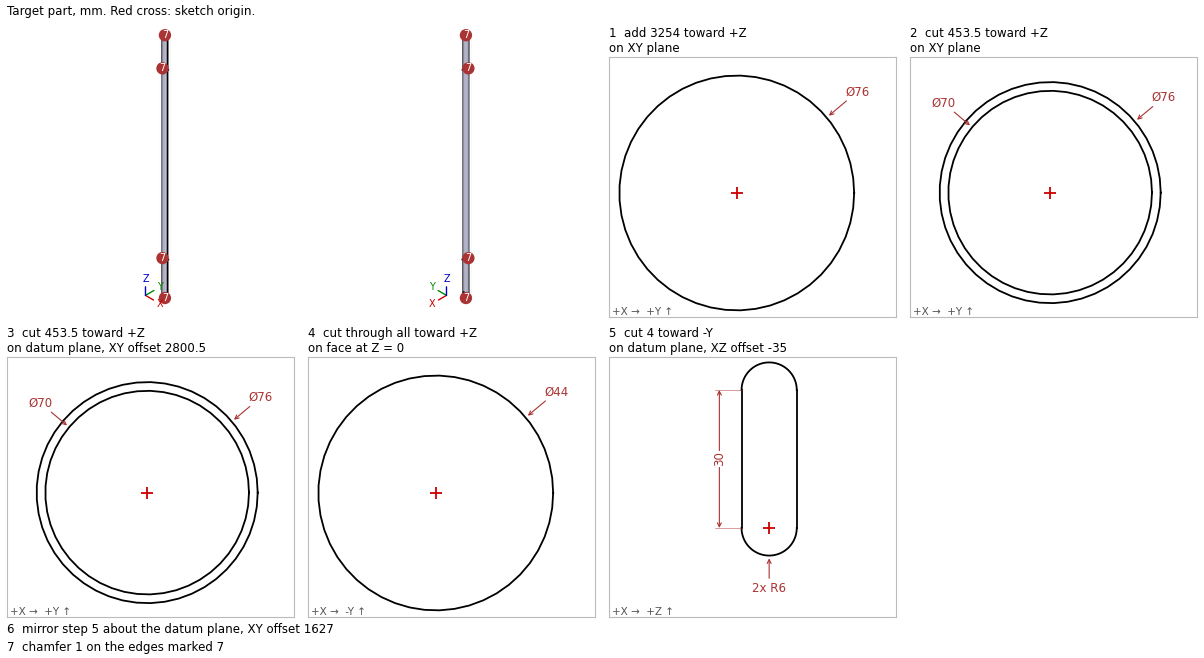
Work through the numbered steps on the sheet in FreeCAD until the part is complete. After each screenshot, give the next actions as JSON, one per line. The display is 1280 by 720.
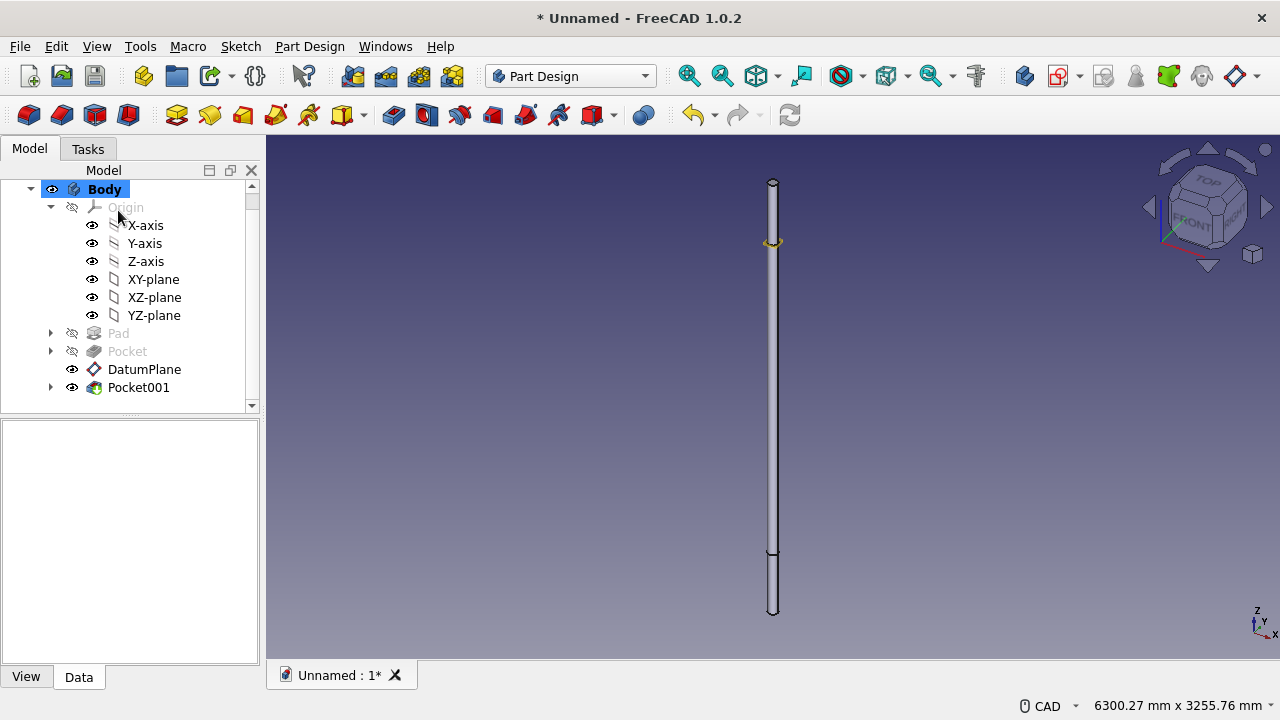
{"action": "left_click", "coordinate": [117, 369]}
{"action": "key", "text": "space"}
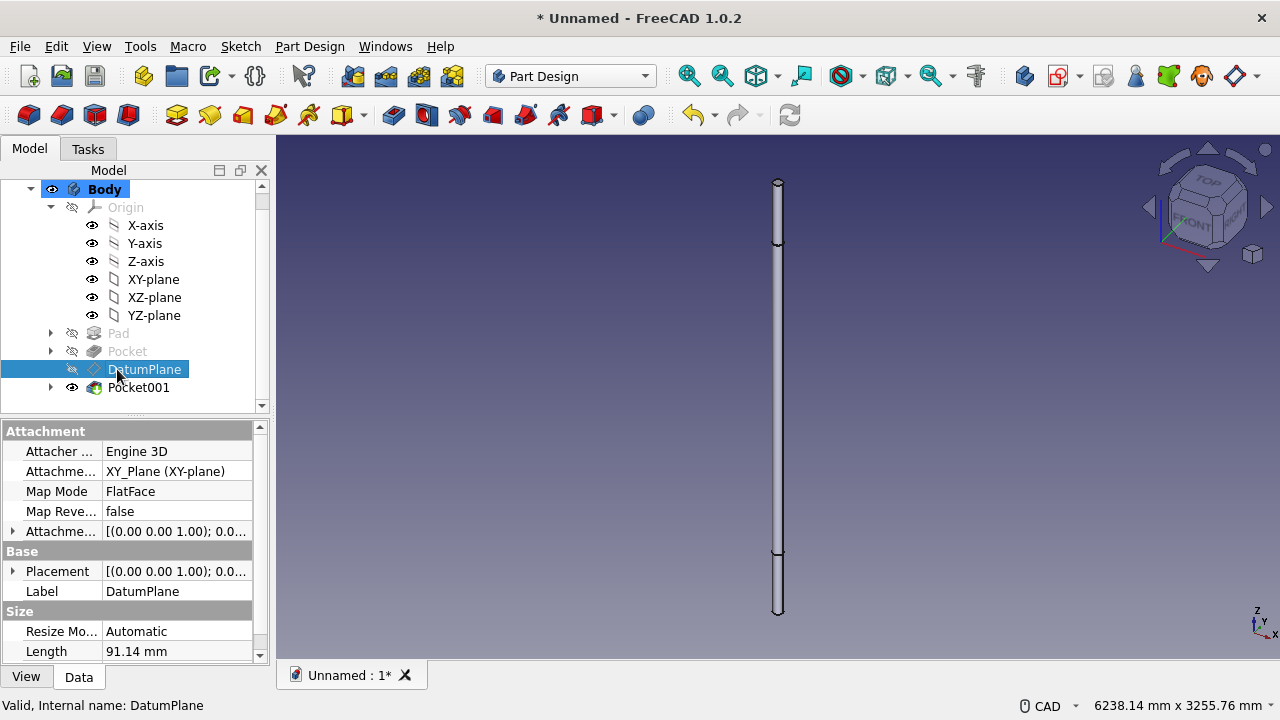
{"action": "key", "text": "5"}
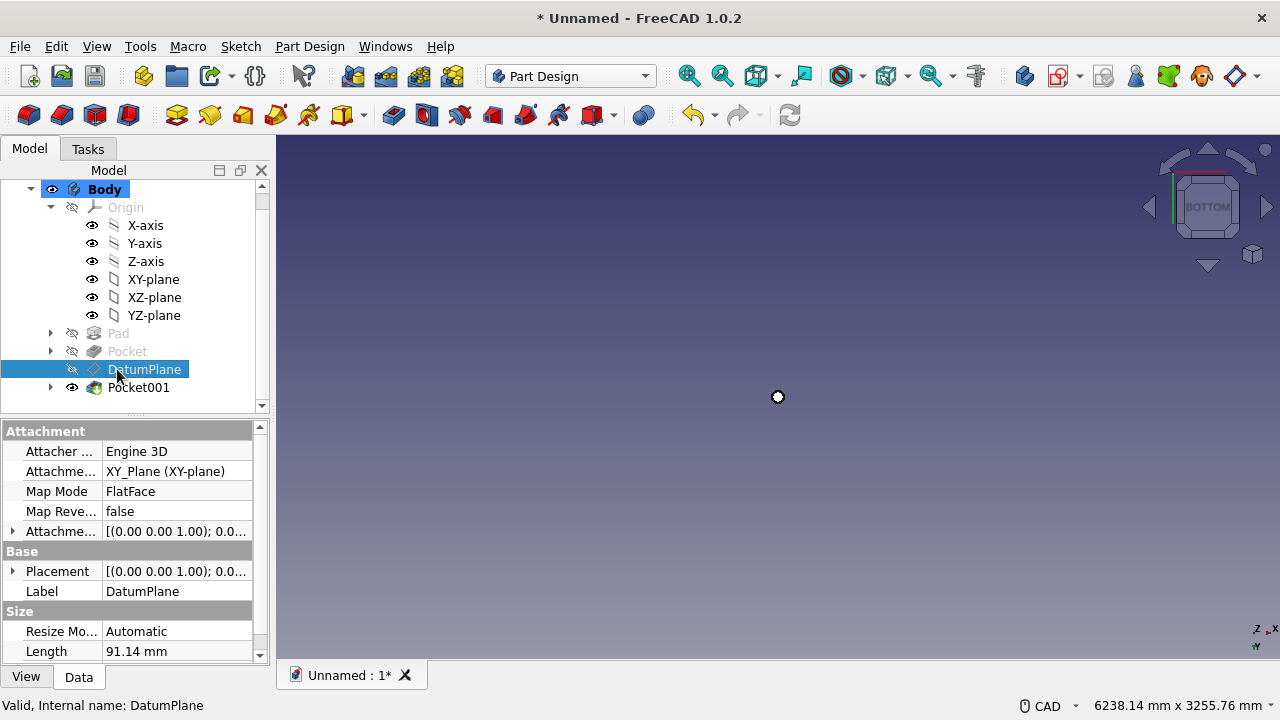
{"action": "left_click", "coordinate": [690, 76]}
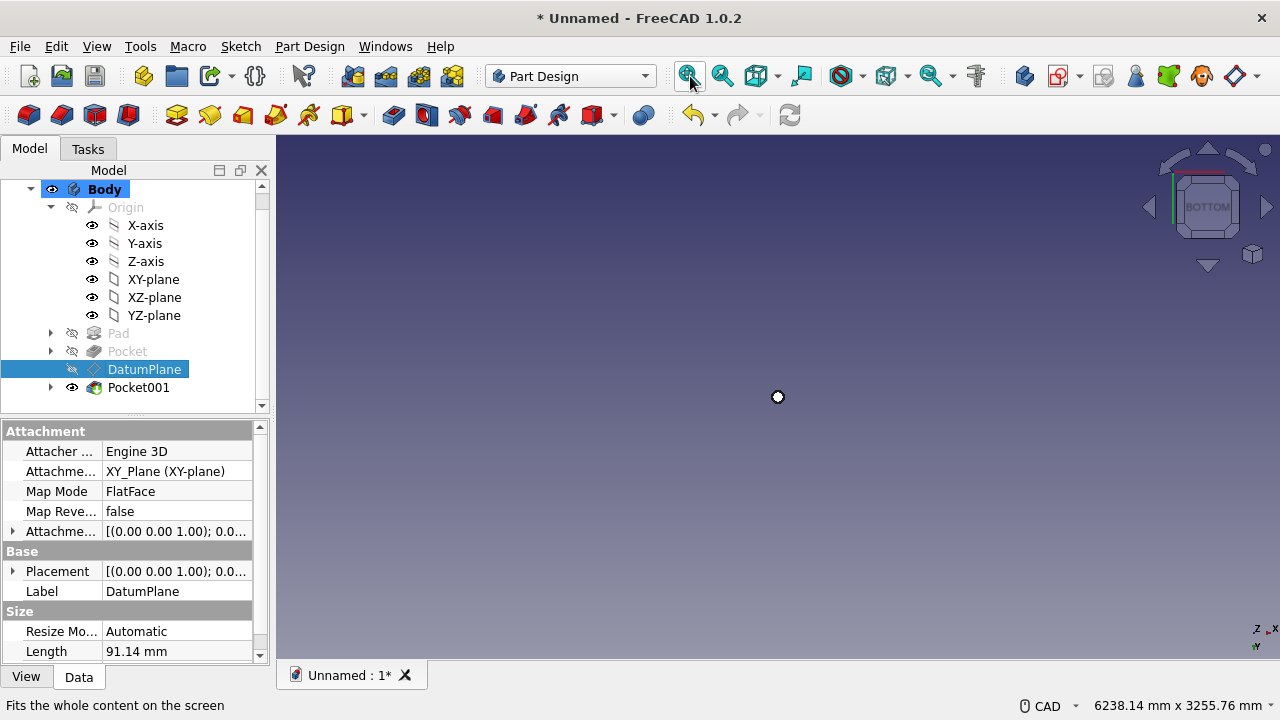
{"action": "scroll", "coordinate": [778, 396], "scroll_direction": "up", "scroll_amount": 4}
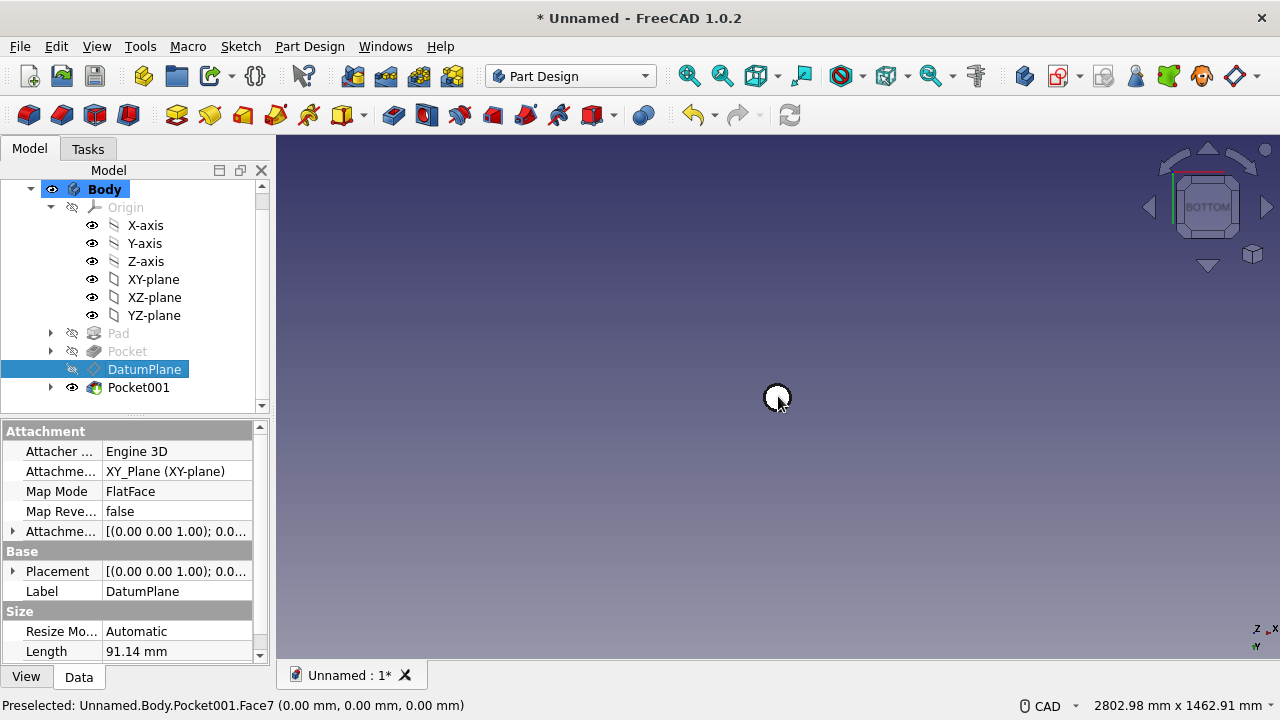
{"action": "left_click", "coordinate": [777, 397]}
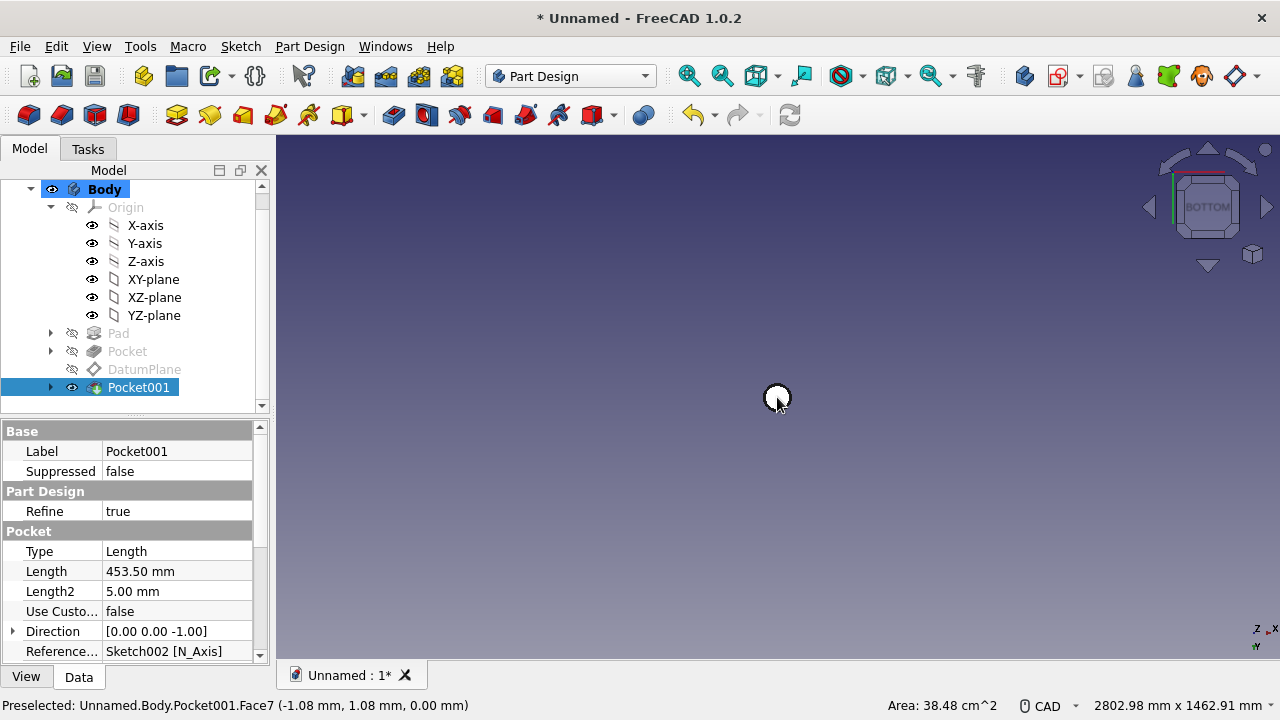
{"action": "left_click", "coordinate": [1058, 76]}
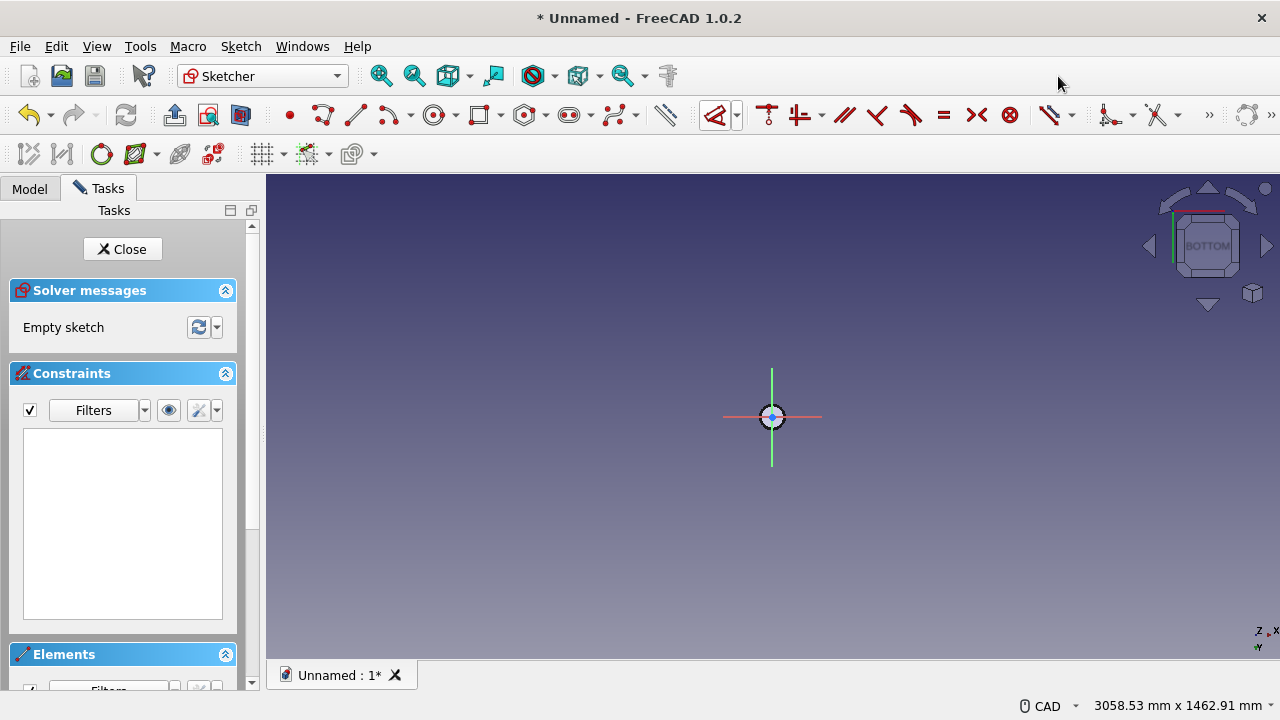
{"action": "scroll", "coordinate": [776, 417], "scroll_direction": "up", "scroll_amount": 15}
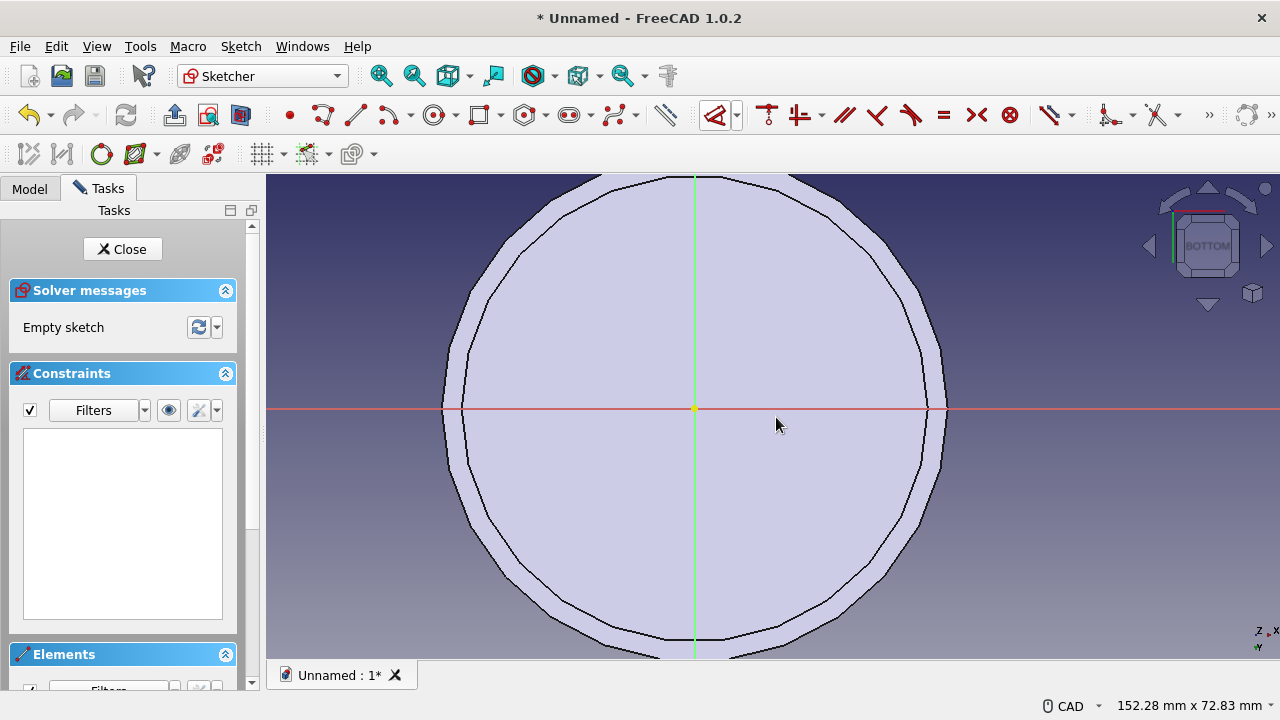
{"action": "left_click", "coordinate": [434, 116]}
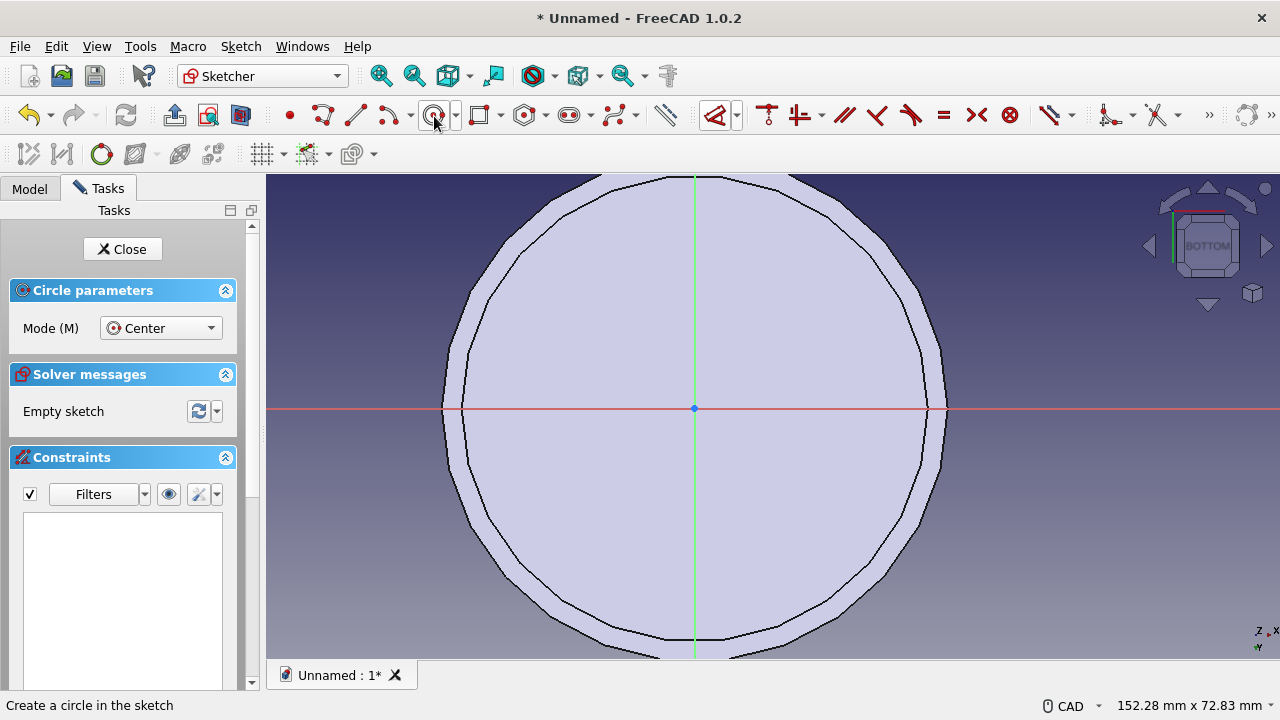
{"action": "left_click", "coordinate": [695, 409]}
{"action": "left_click", "coordinate": [798, 305]}
{"action": "key", "text": "Escape"}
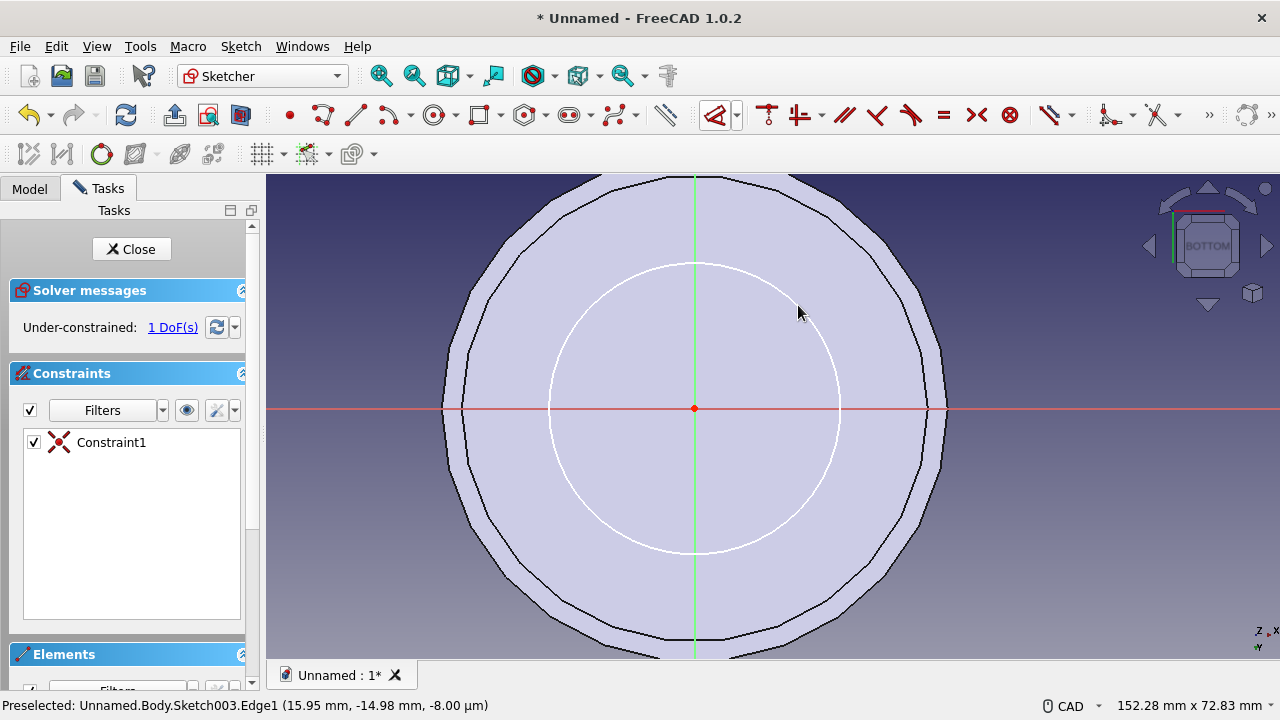
{"action": "left_click", "coordinate": [797, 305]}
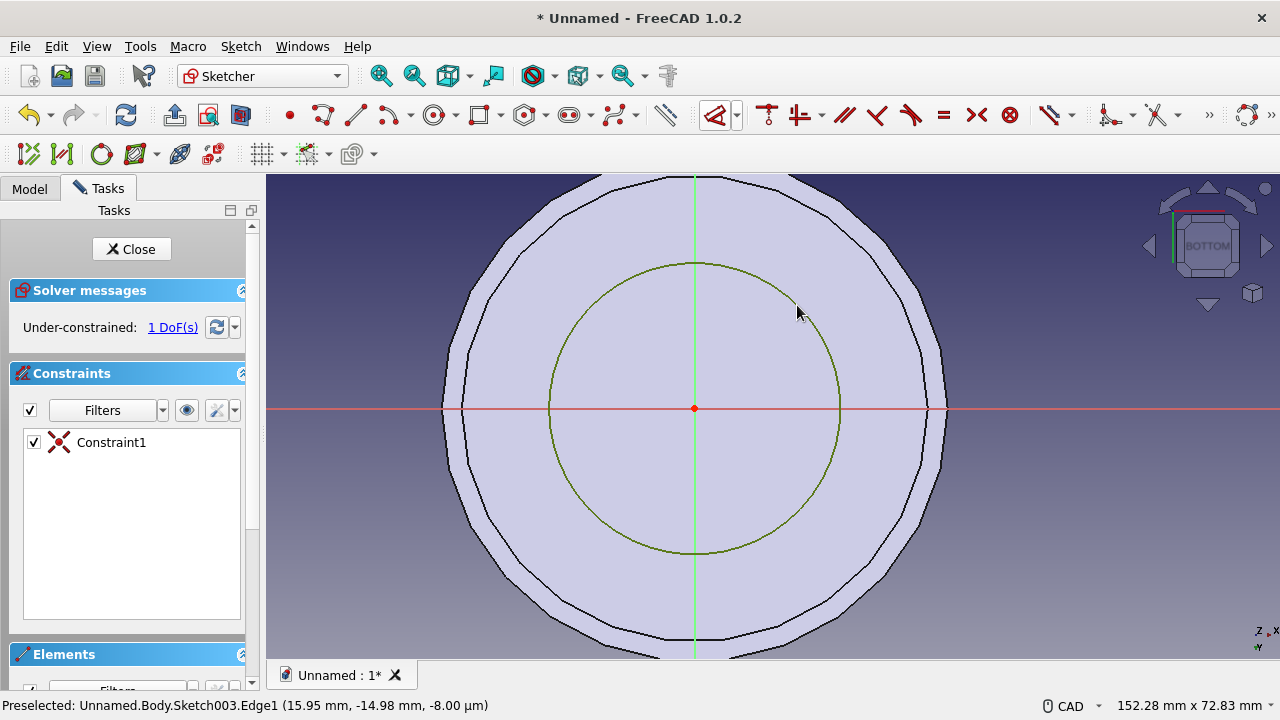
{"action": "key", "text": "k o"}